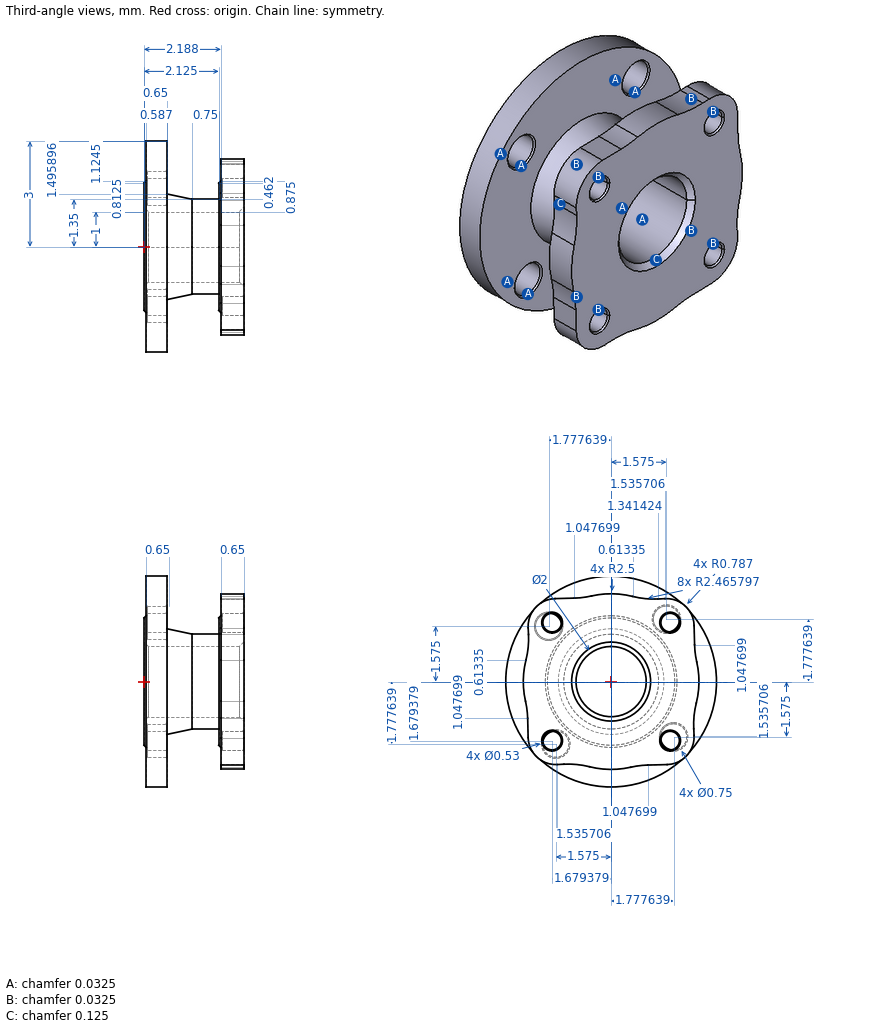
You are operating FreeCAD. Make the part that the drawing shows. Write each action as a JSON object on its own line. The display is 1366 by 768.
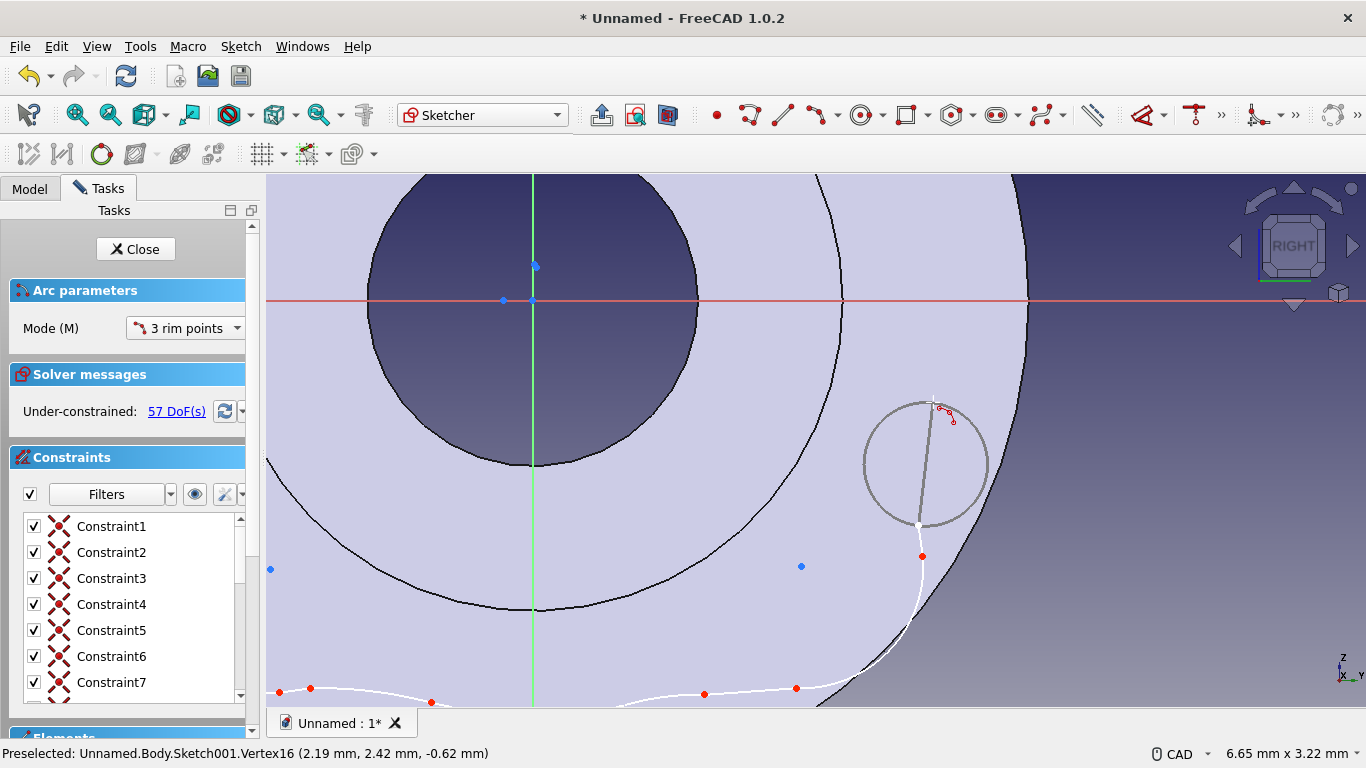
{"action": "scroll", "coordinate": [923, 462], "scroll_direction": "up", "scroll_amount": 7}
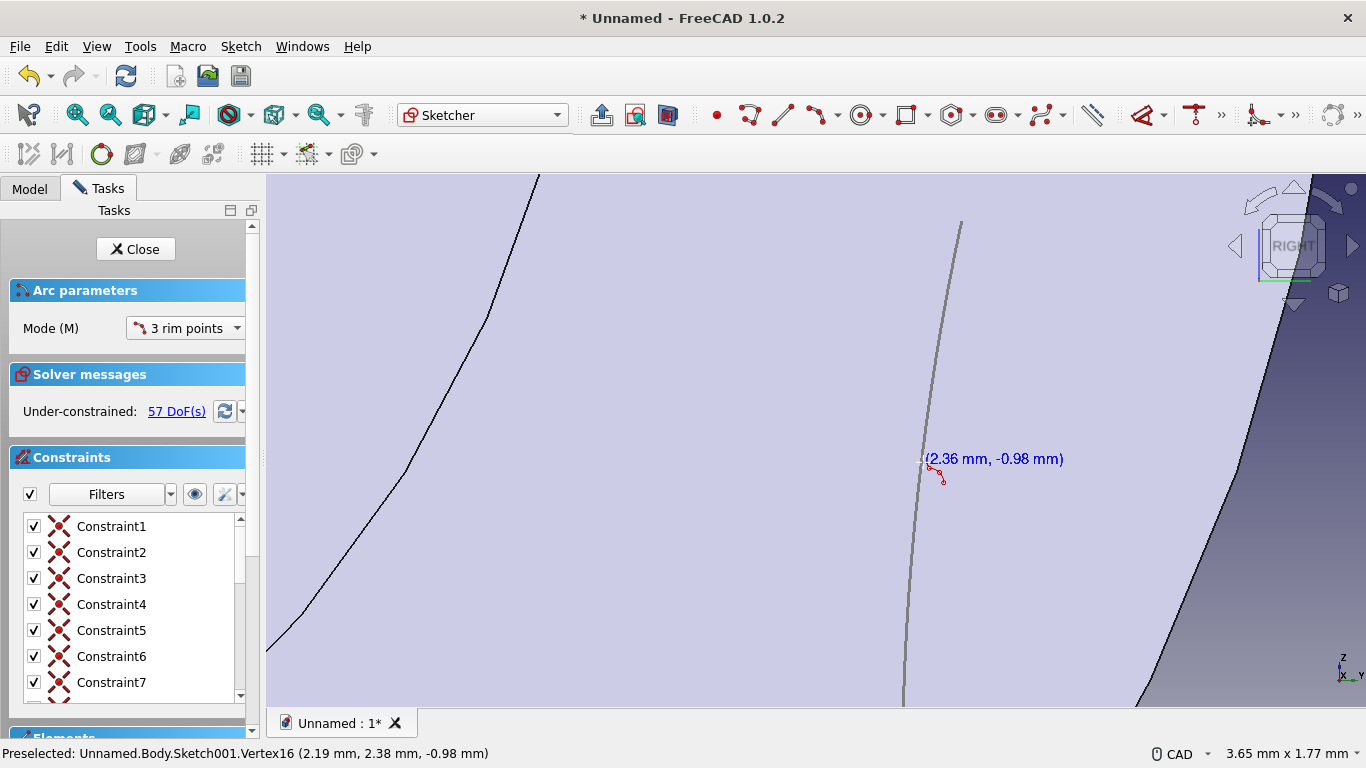
{"action": "left_click", "coordinate": [921, 461]}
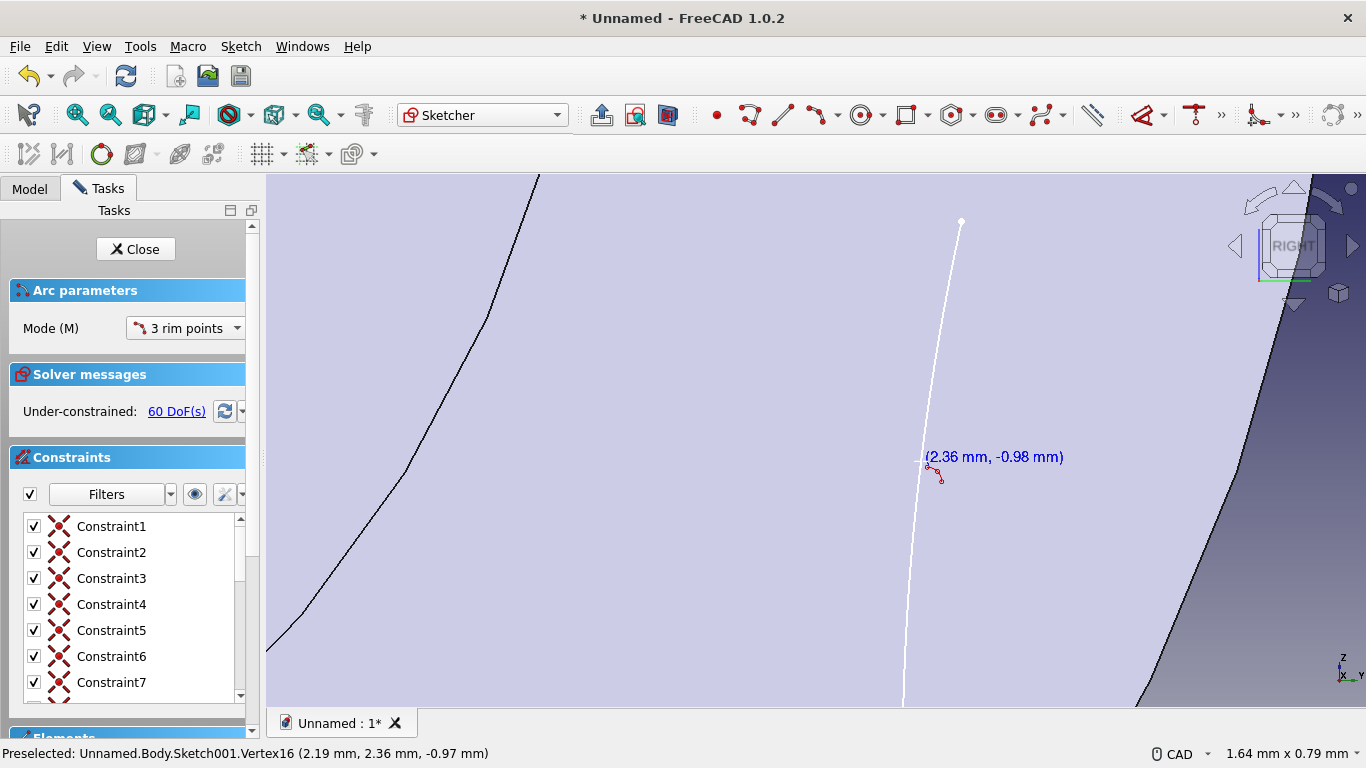
{"action": "scroll", "coordinate": [923, 519], "scroll_direction": "down", "scroll_amount": 11}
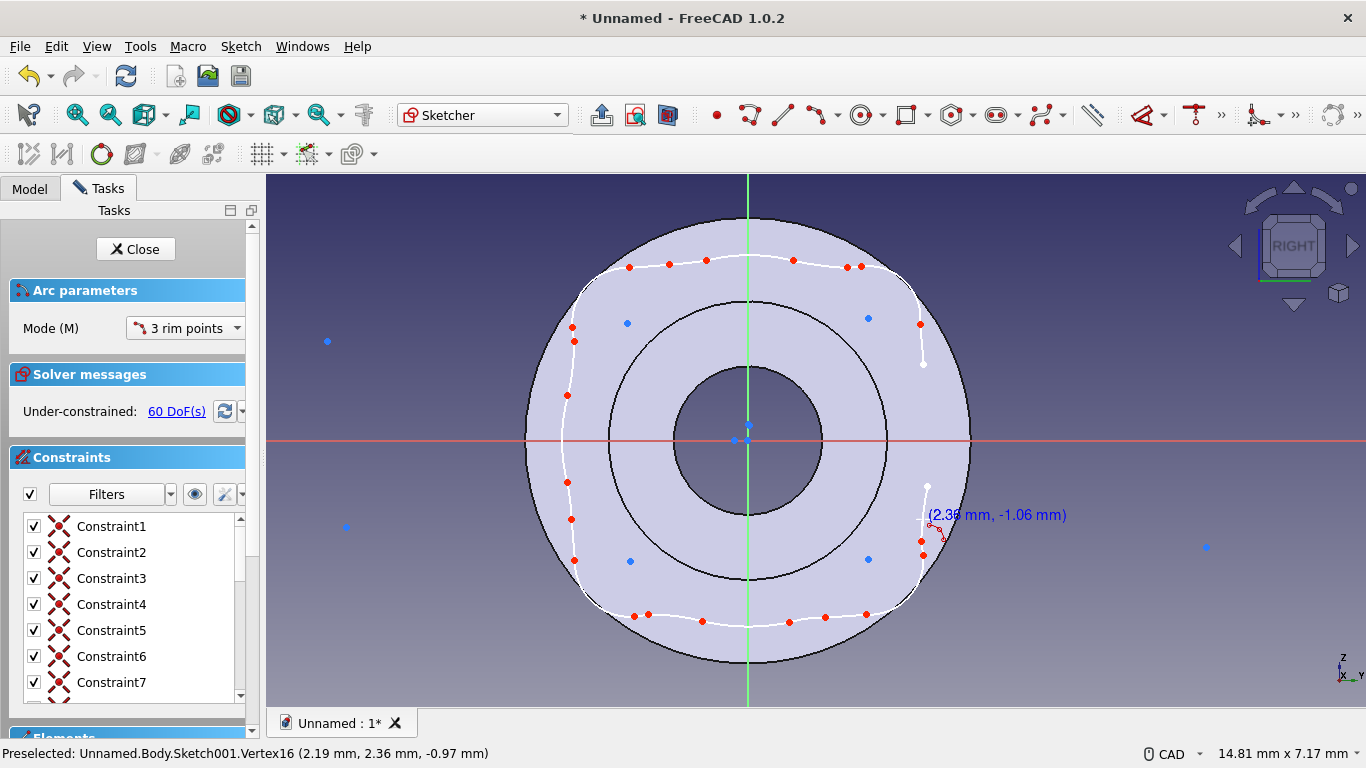
{"action": "left_click", "coordinate": [928, 487]}
{"action": "left_click", "coordinate": [929, 399]}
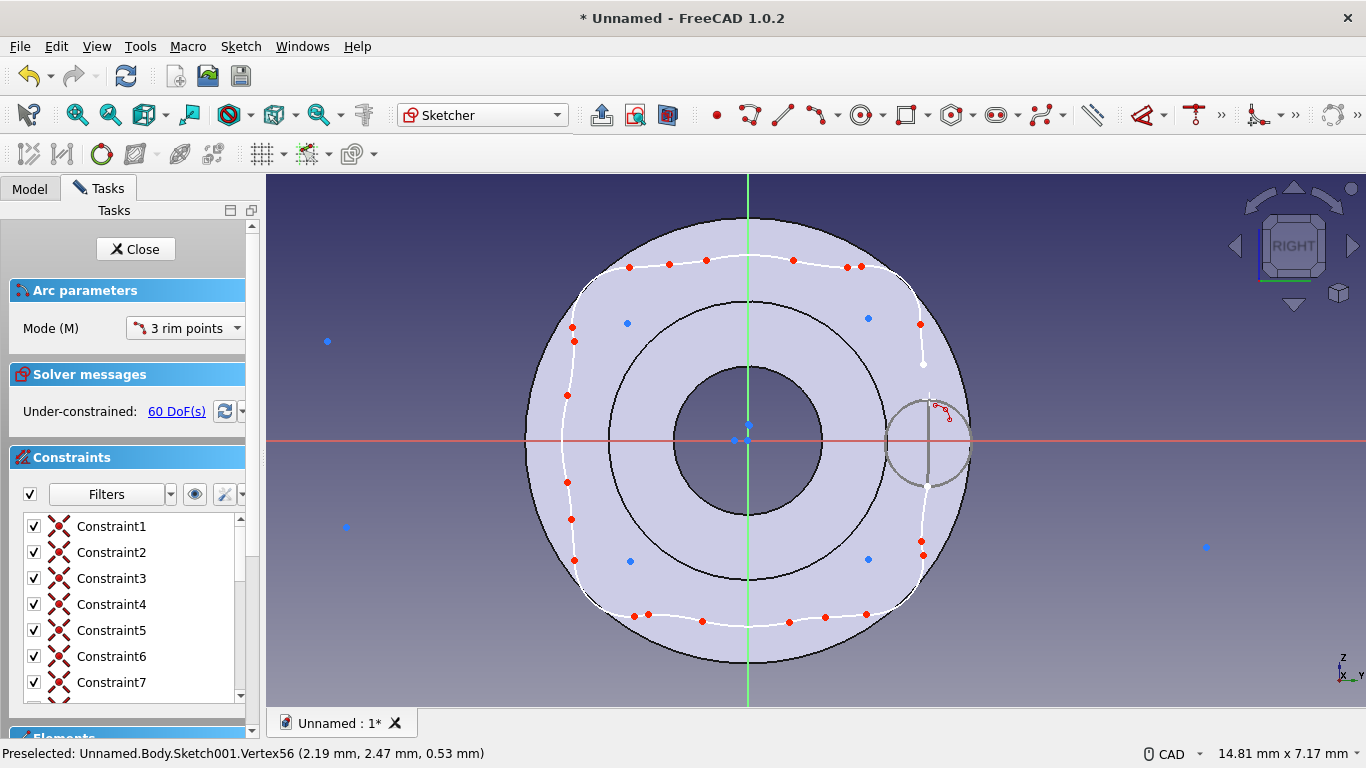
{"action": "scroll", "coordinate": [934, 434], "scroll_direction": "up", "scroll_amount": 6}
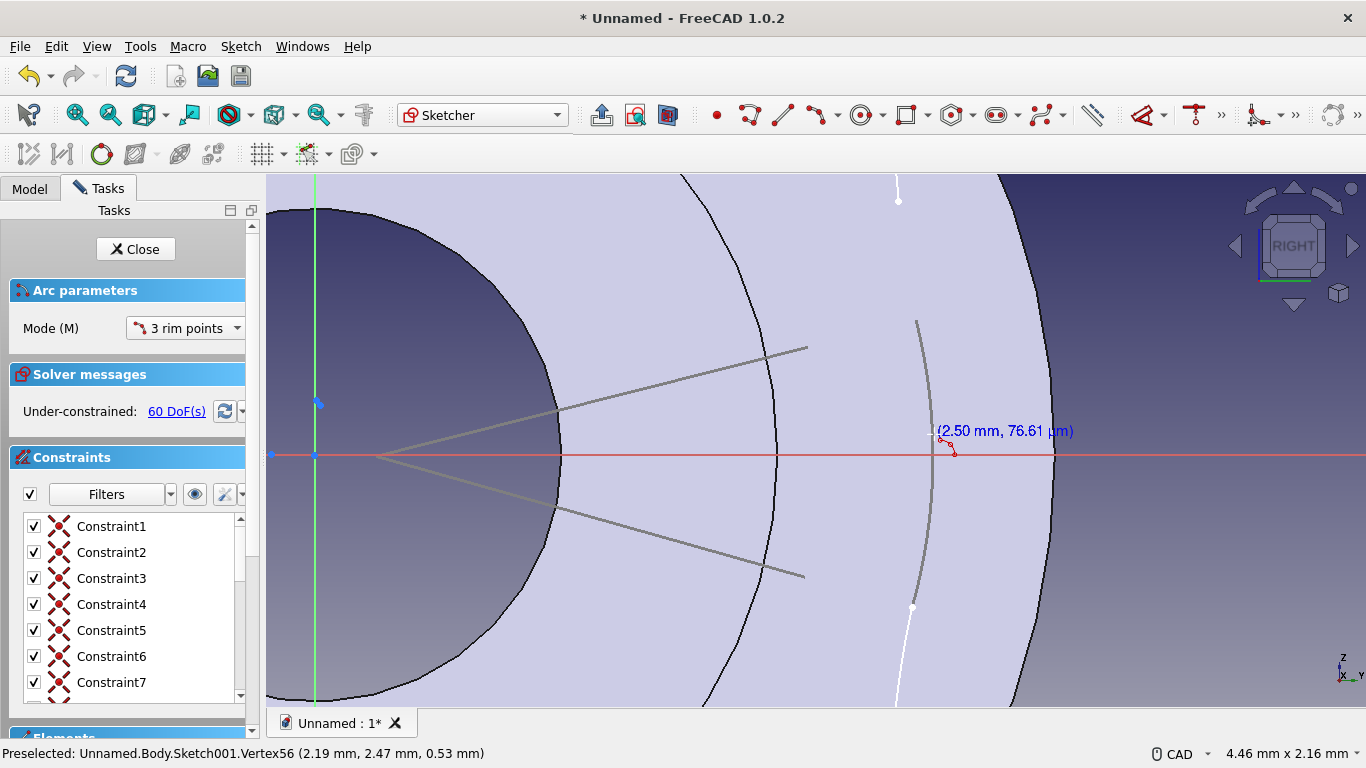
{"action": "left_click", "coordinate": [931, 433]}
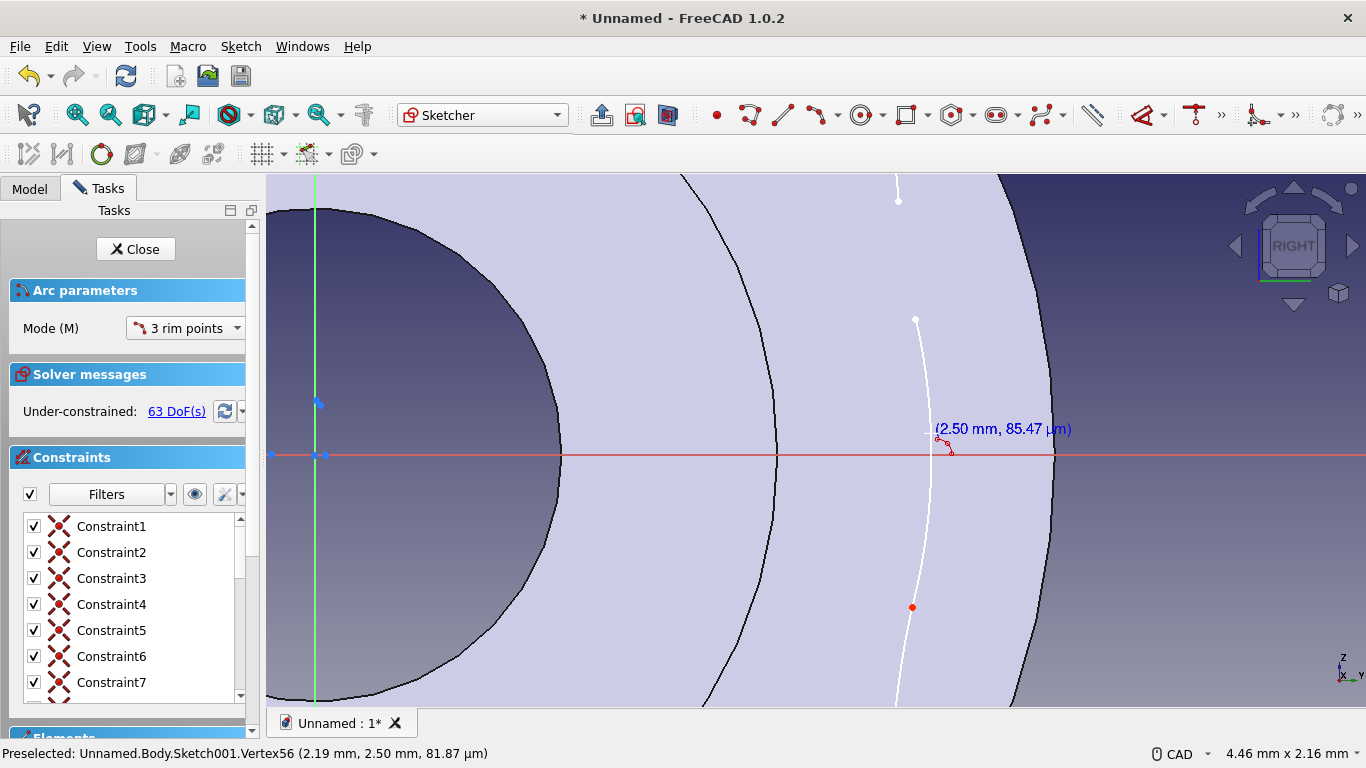
{"action": "scroll", "coordinate": [934, 434], "scroll_direction": "down", "scroll_amount": 6}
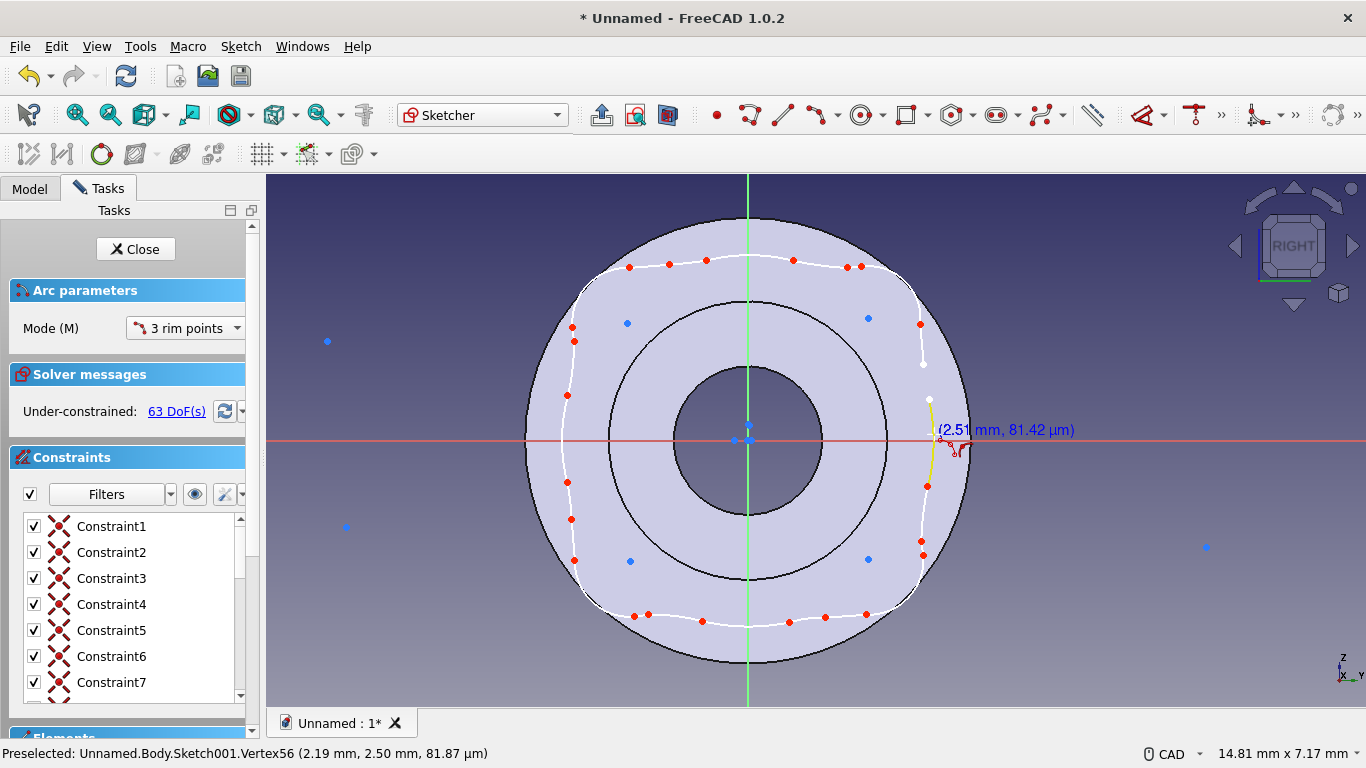
{"action": "left_click", "coordinate": [929, 400]}
{"action": "left_click", "coordinate": [924, 364]}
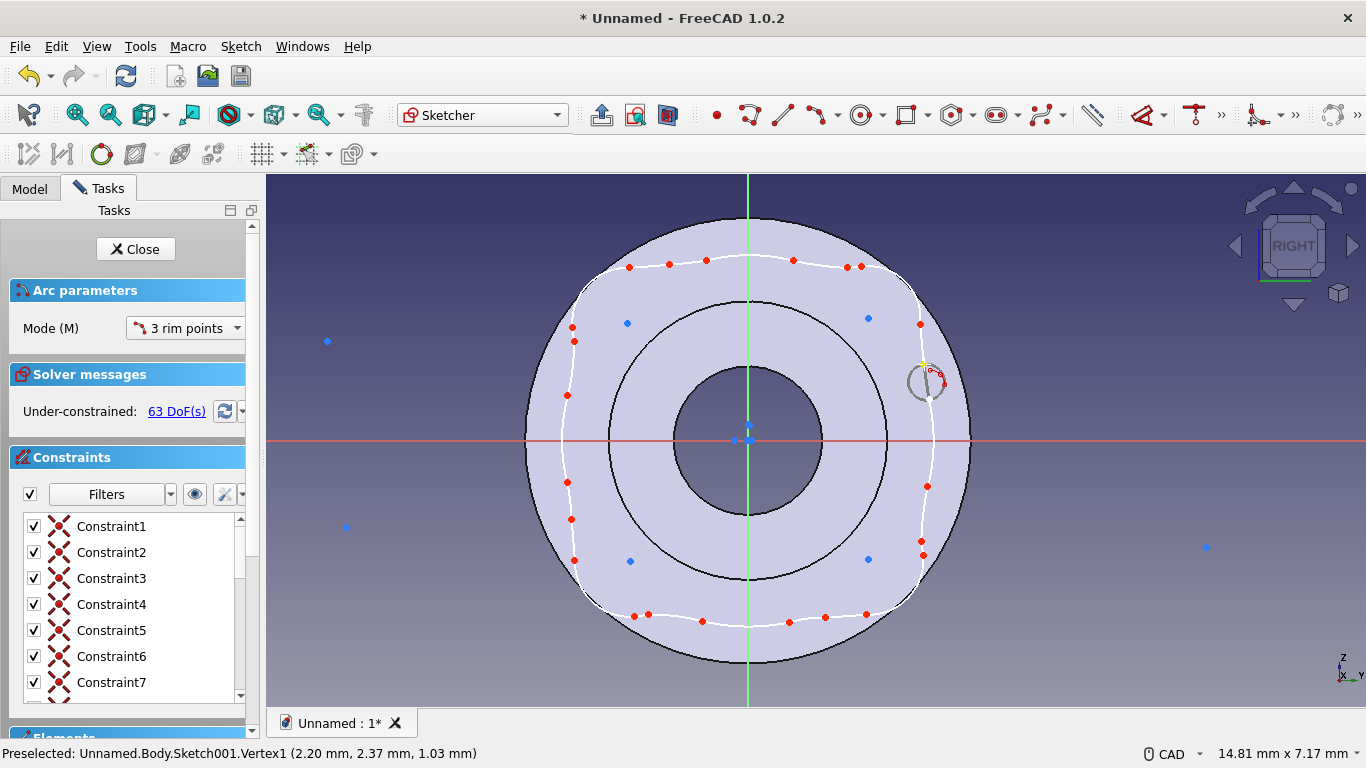
{"action": "scroll", "coordinate": [926, 381], "scroll_direction": "up", "scroll_amount": 15}